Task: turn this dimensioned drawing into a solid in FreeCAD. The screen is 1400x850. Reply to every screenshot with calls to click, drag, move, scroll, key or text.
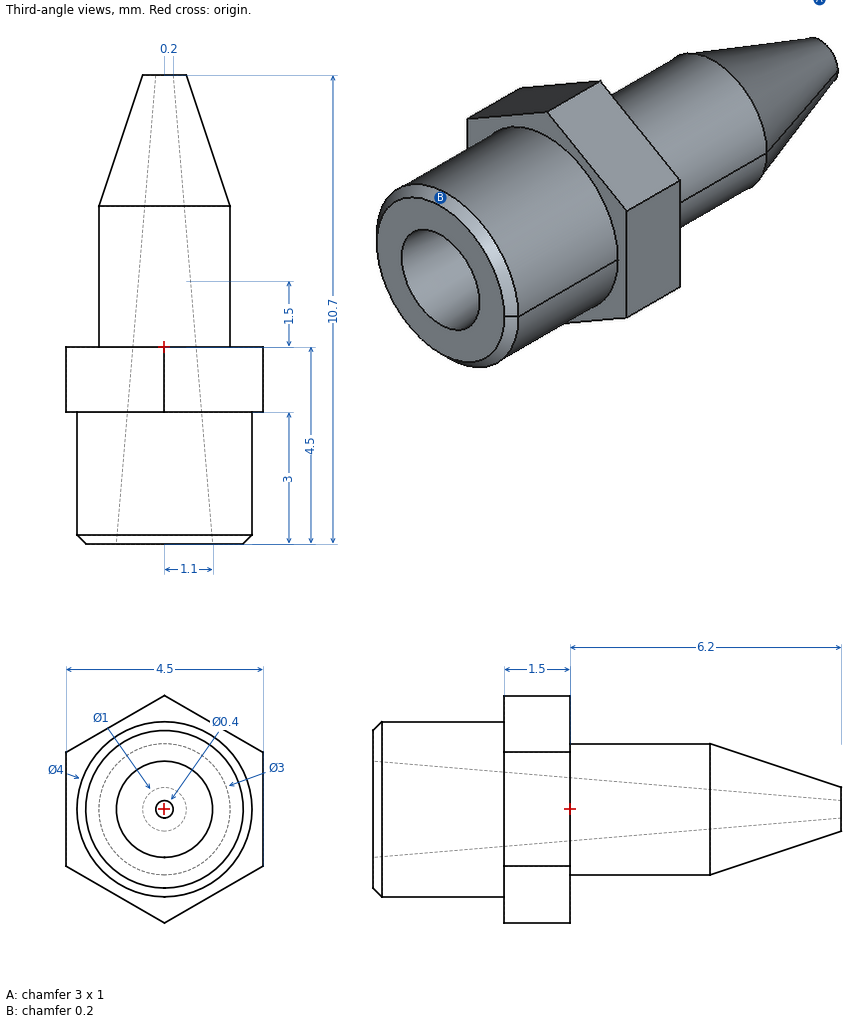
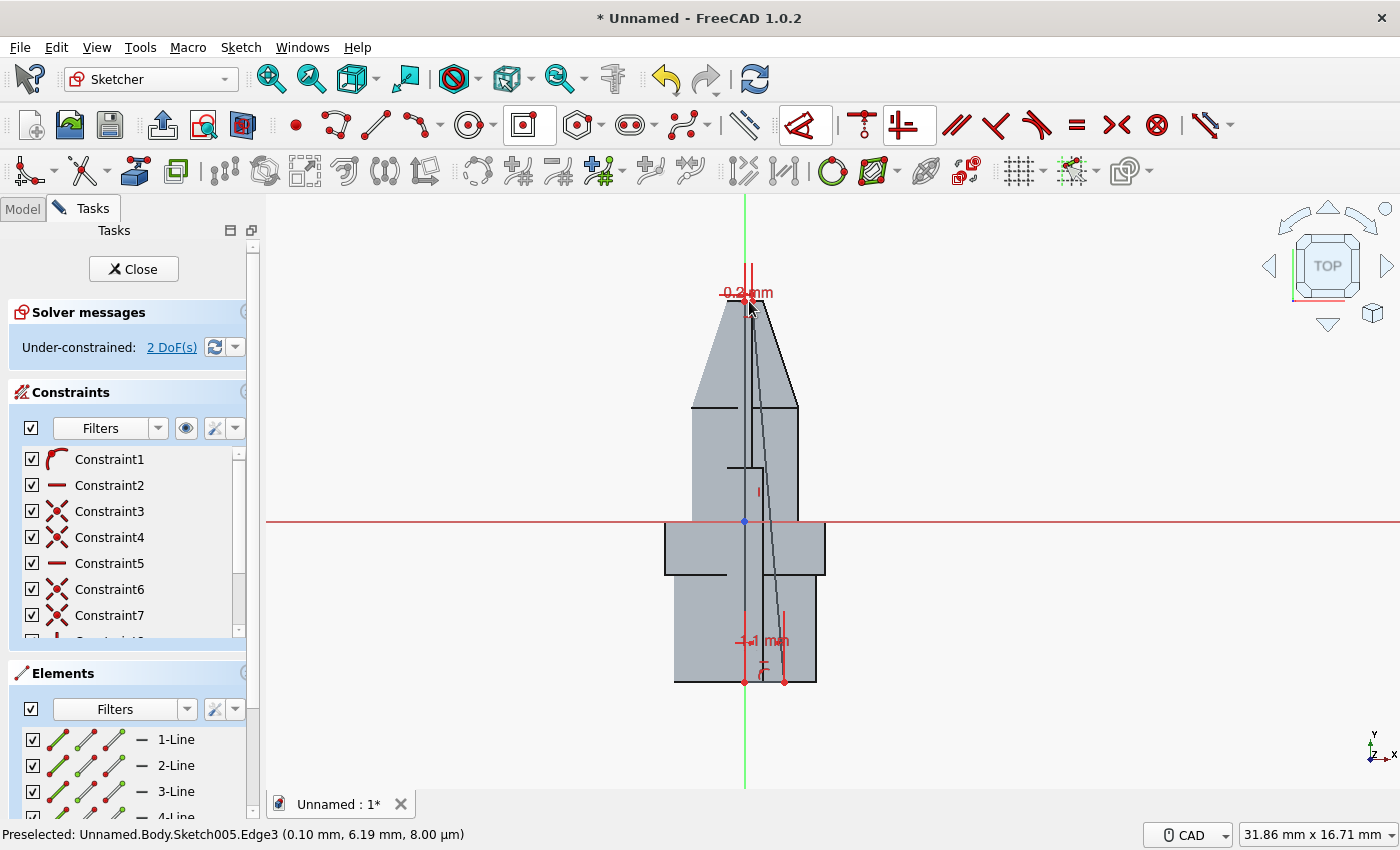
click(745, 416)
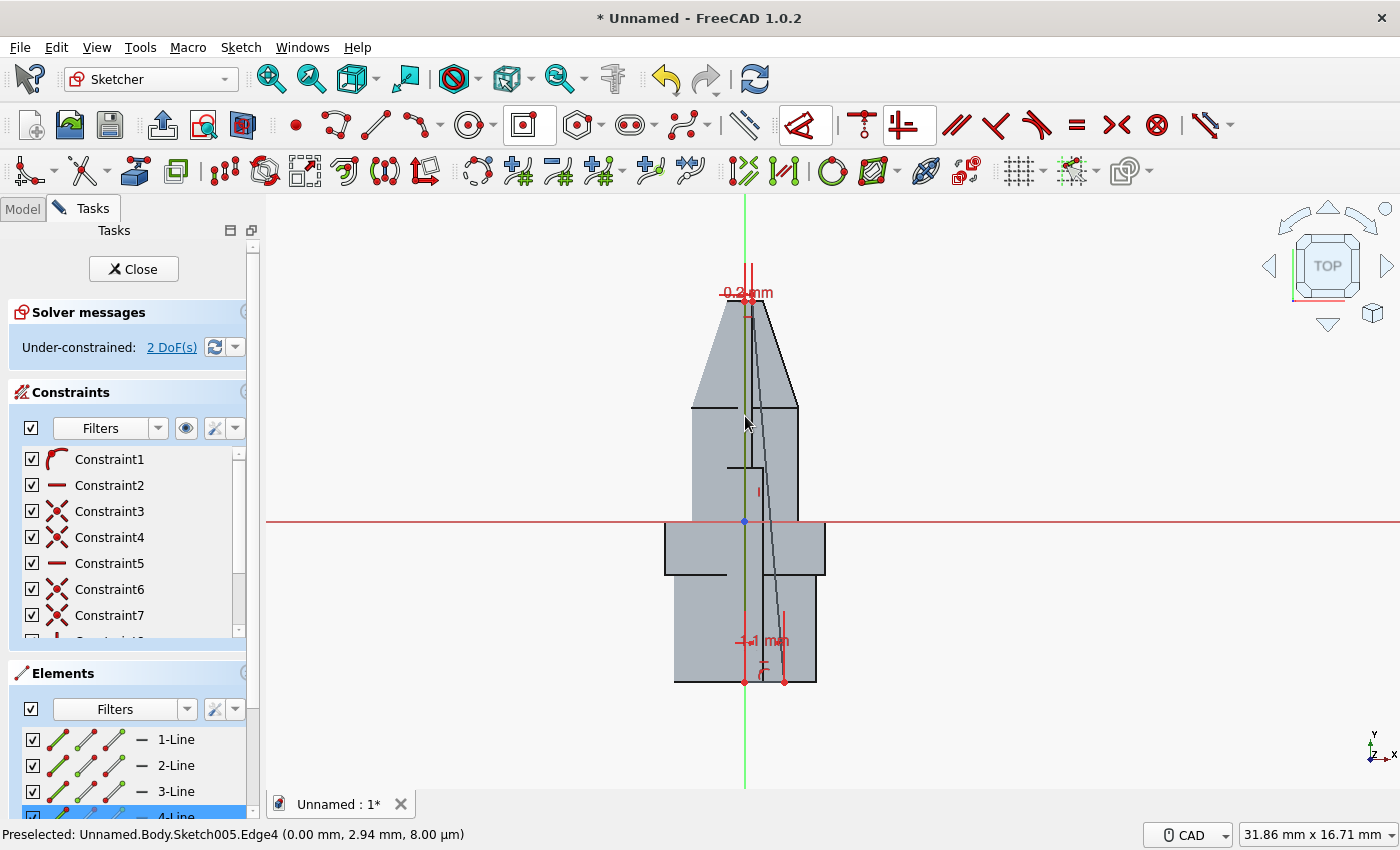
key(i)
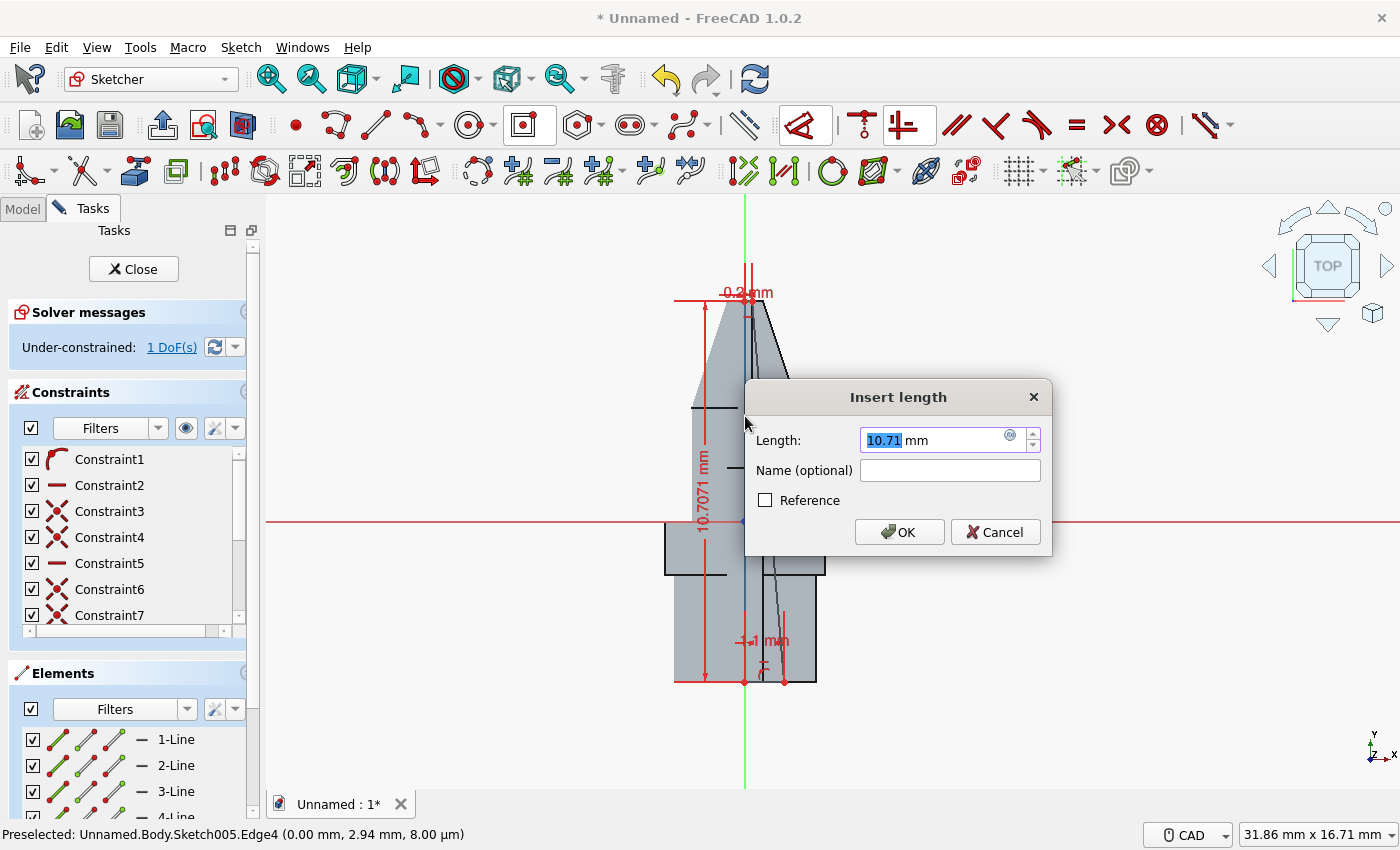
text(10.7)
key(Return)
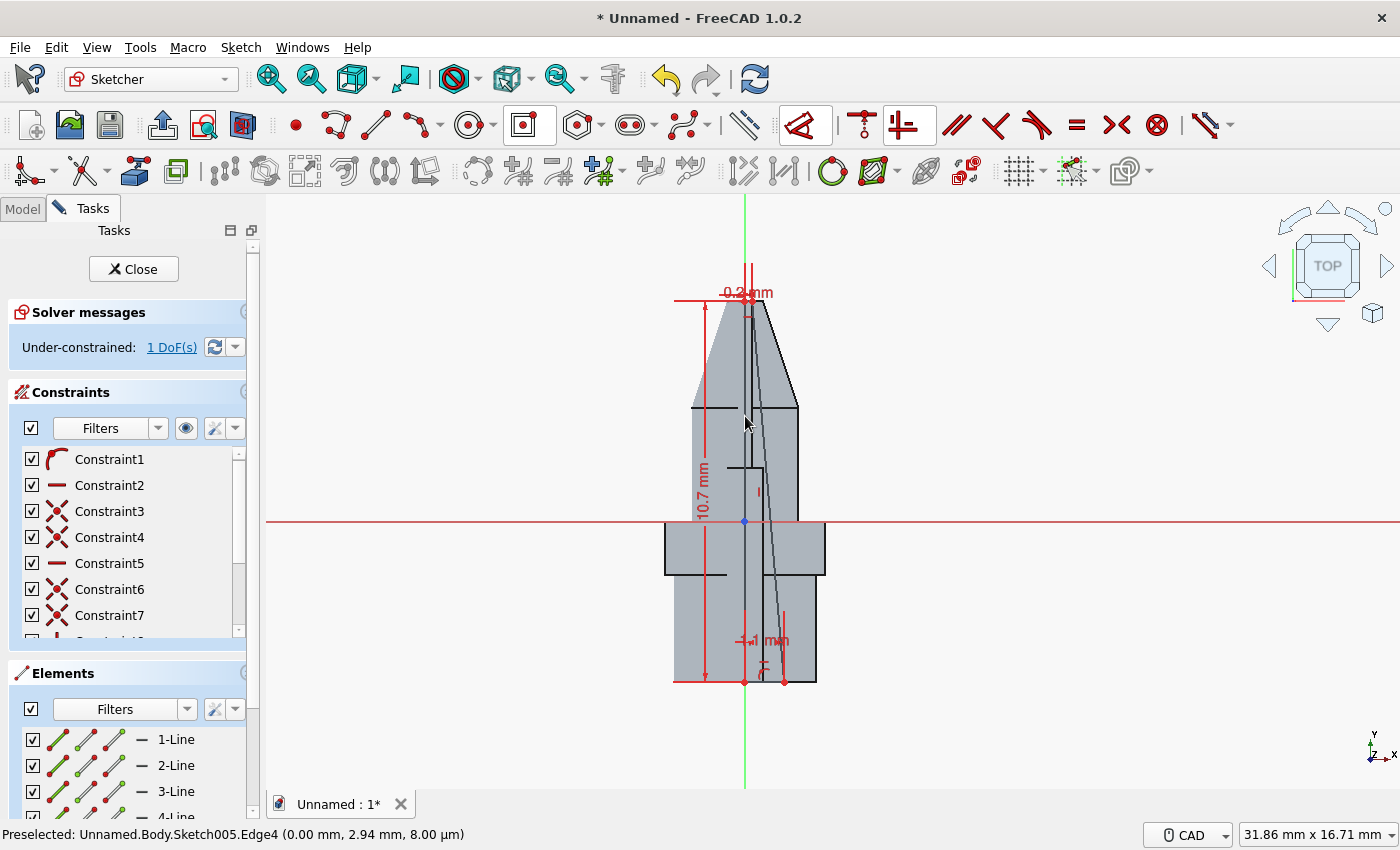
click(745, 682)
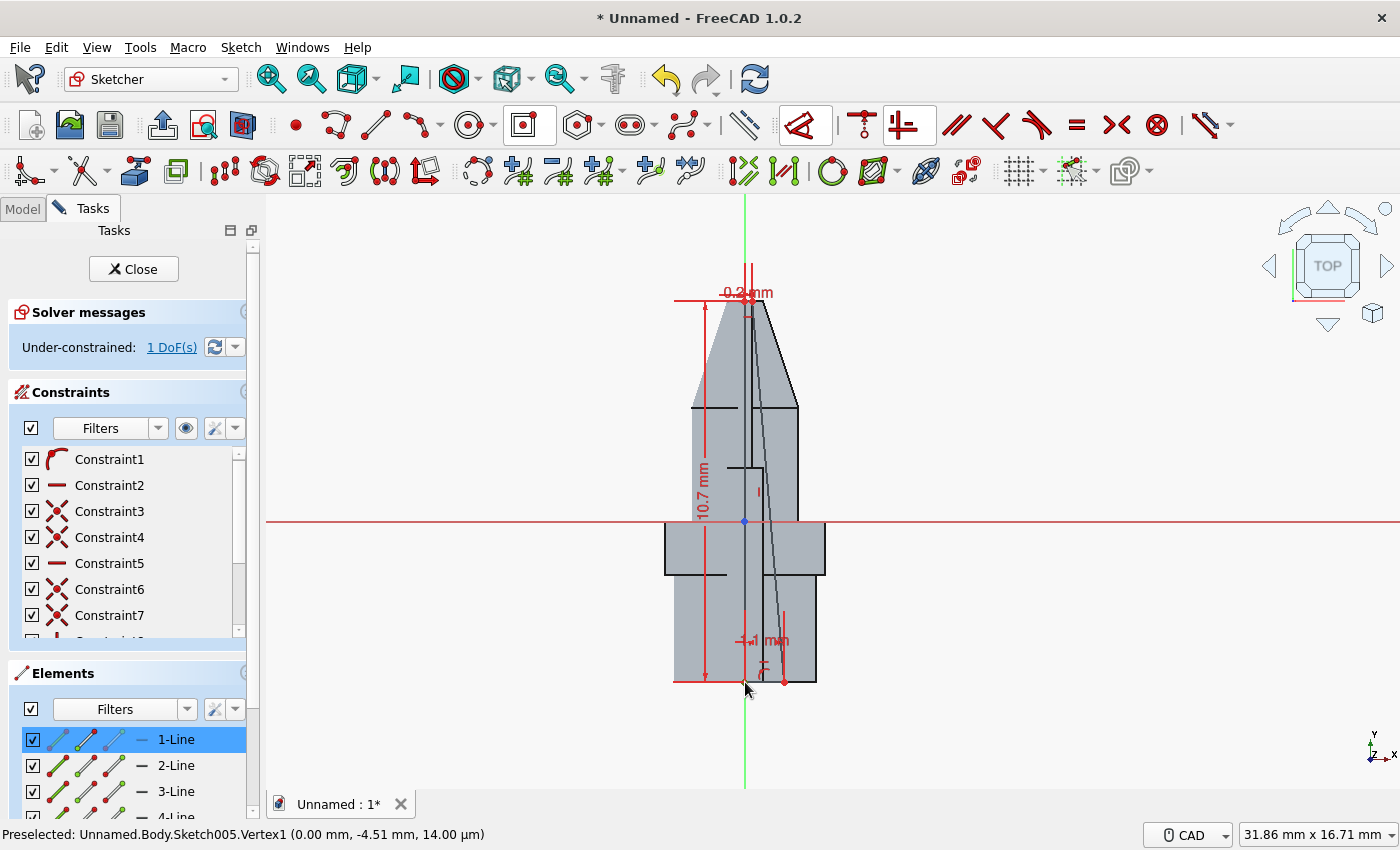
key(i)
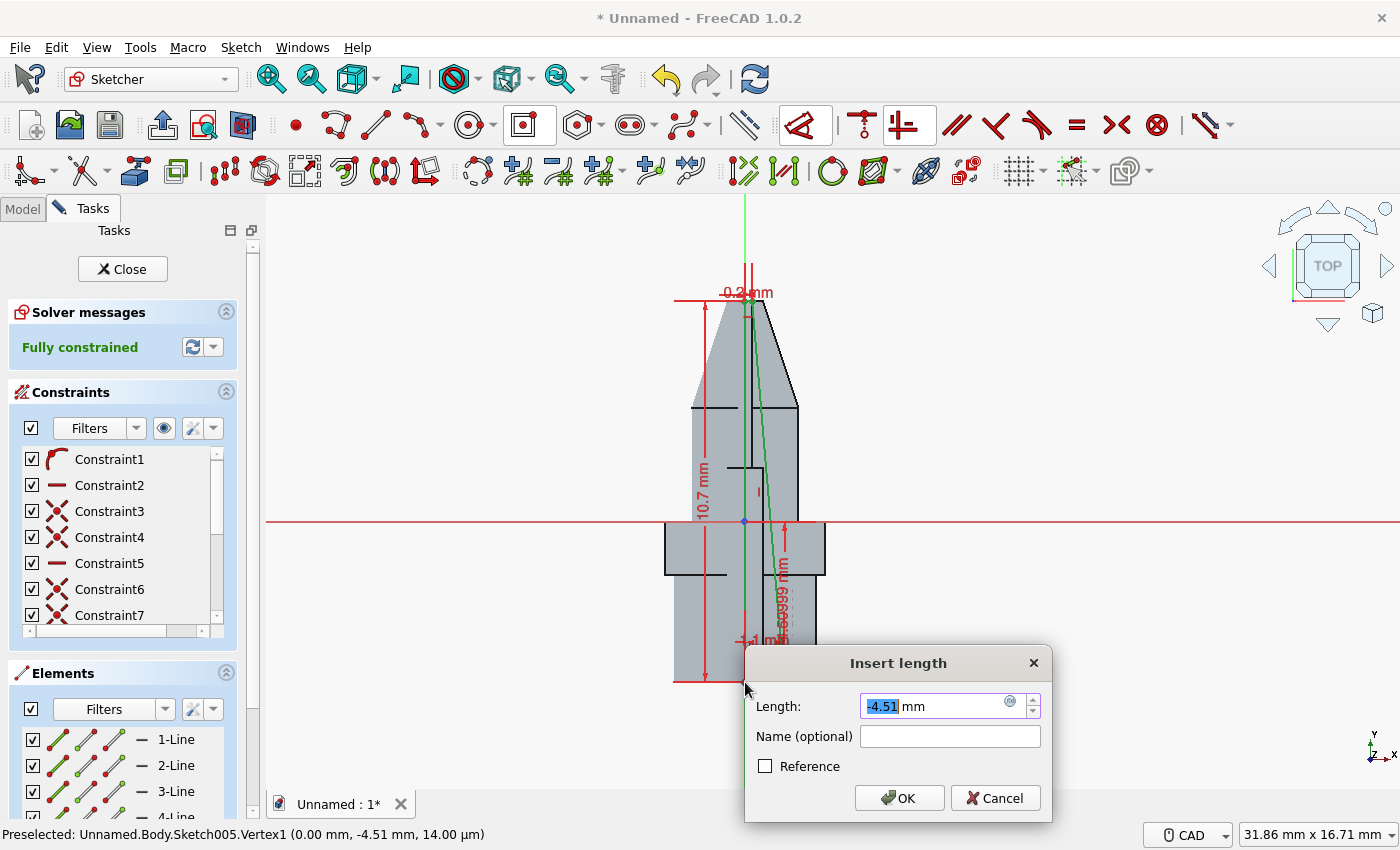
text(-4.5)
key(Return)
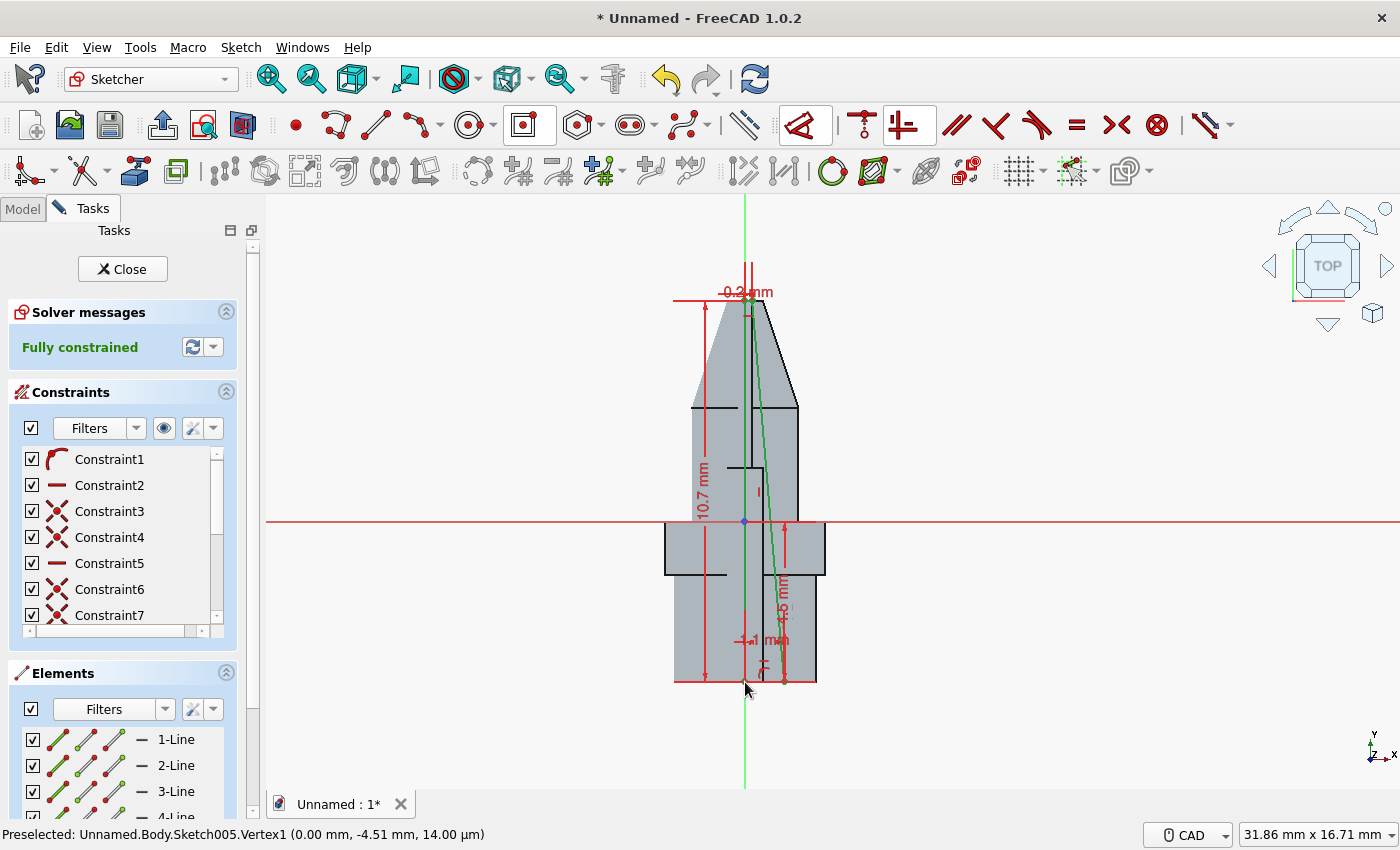
click(123, 269)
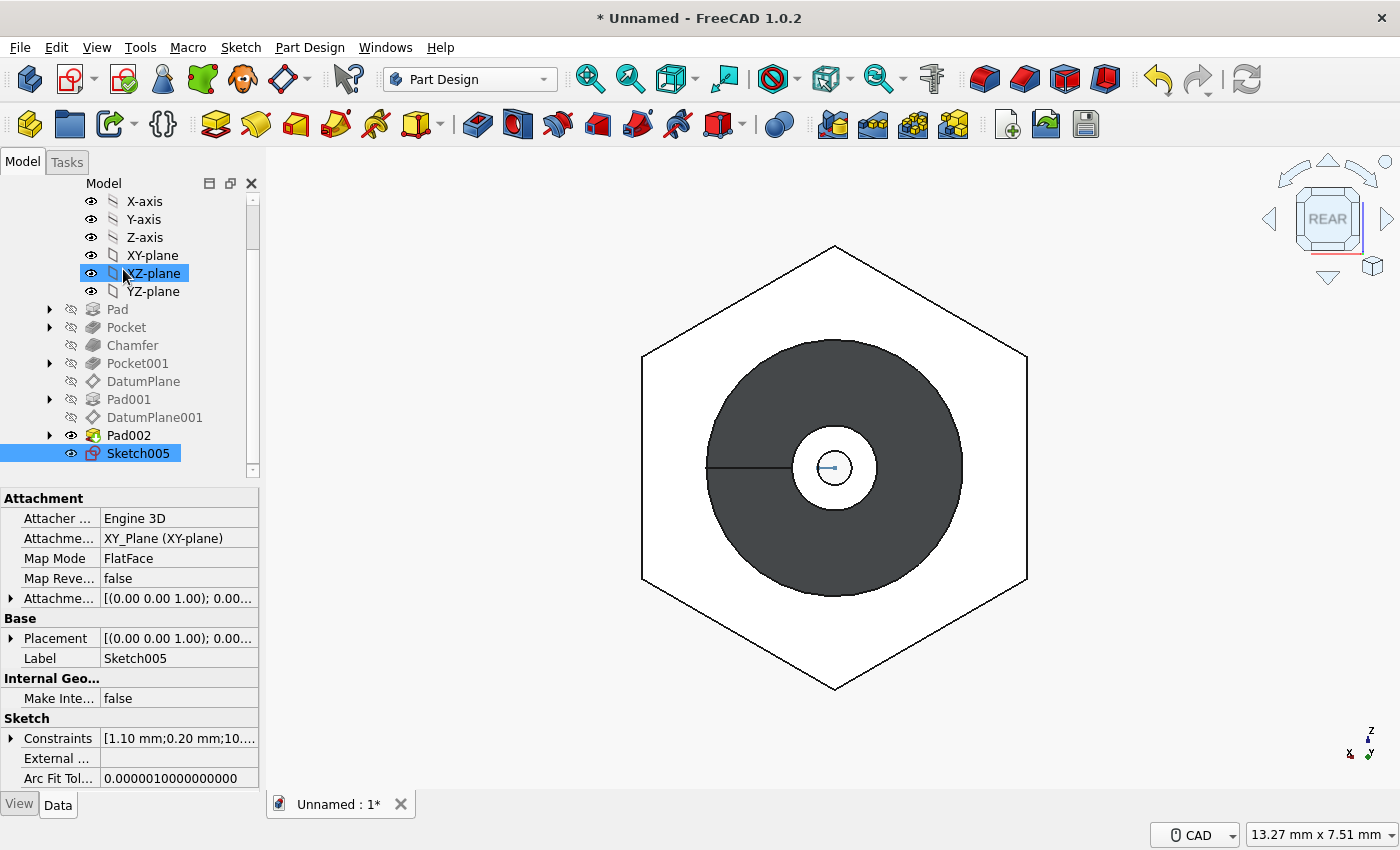
click(558, 124)